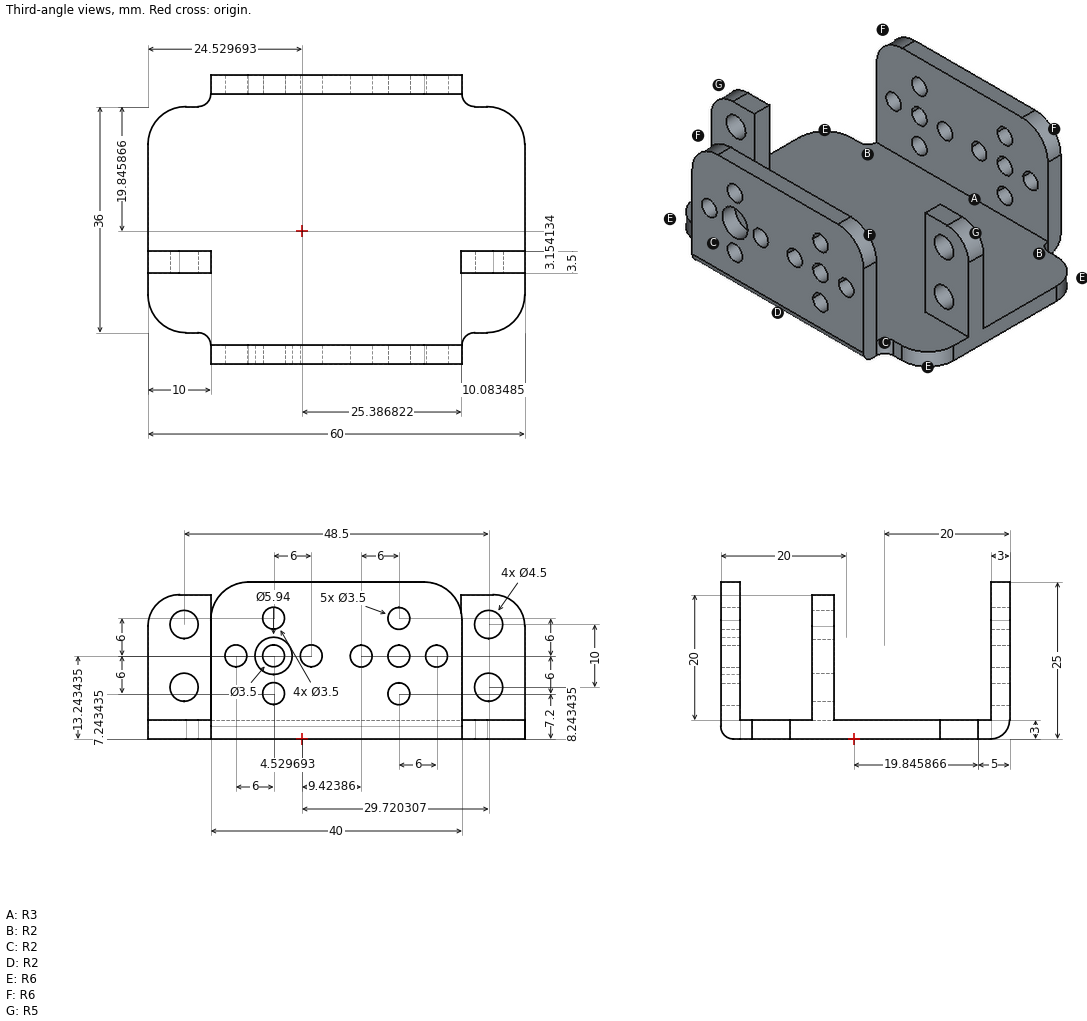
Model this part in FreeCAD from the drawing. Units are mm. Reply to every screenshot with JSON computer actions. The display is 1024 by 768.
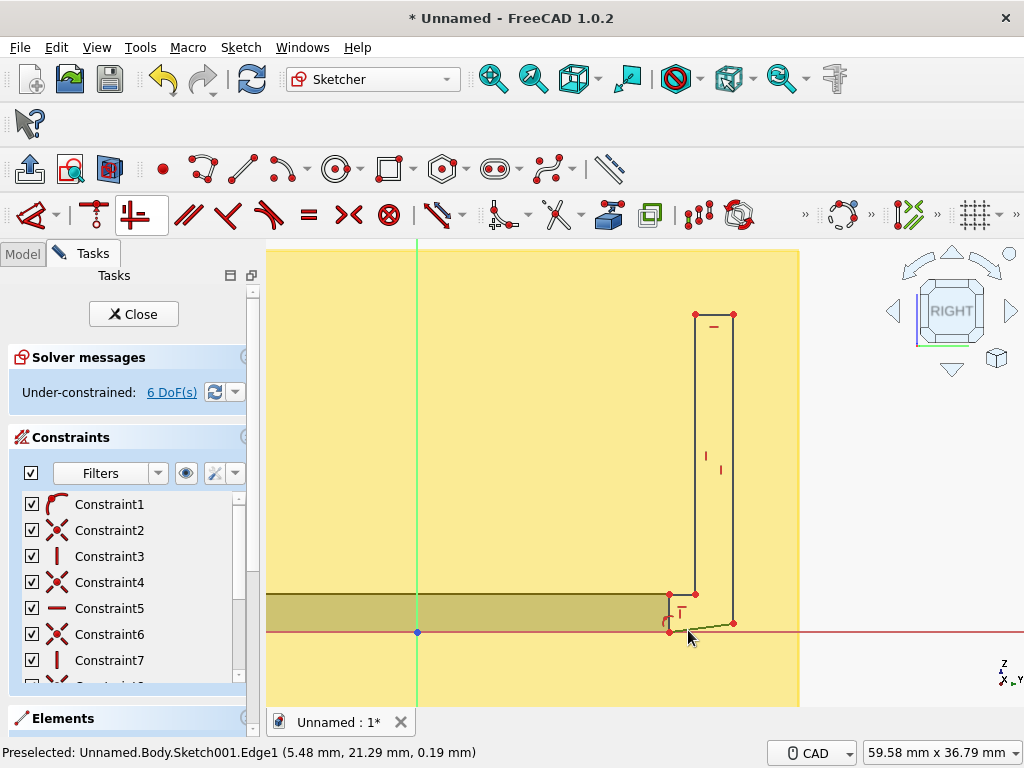
{"action": "left_click", "coordinate": [162, 216]}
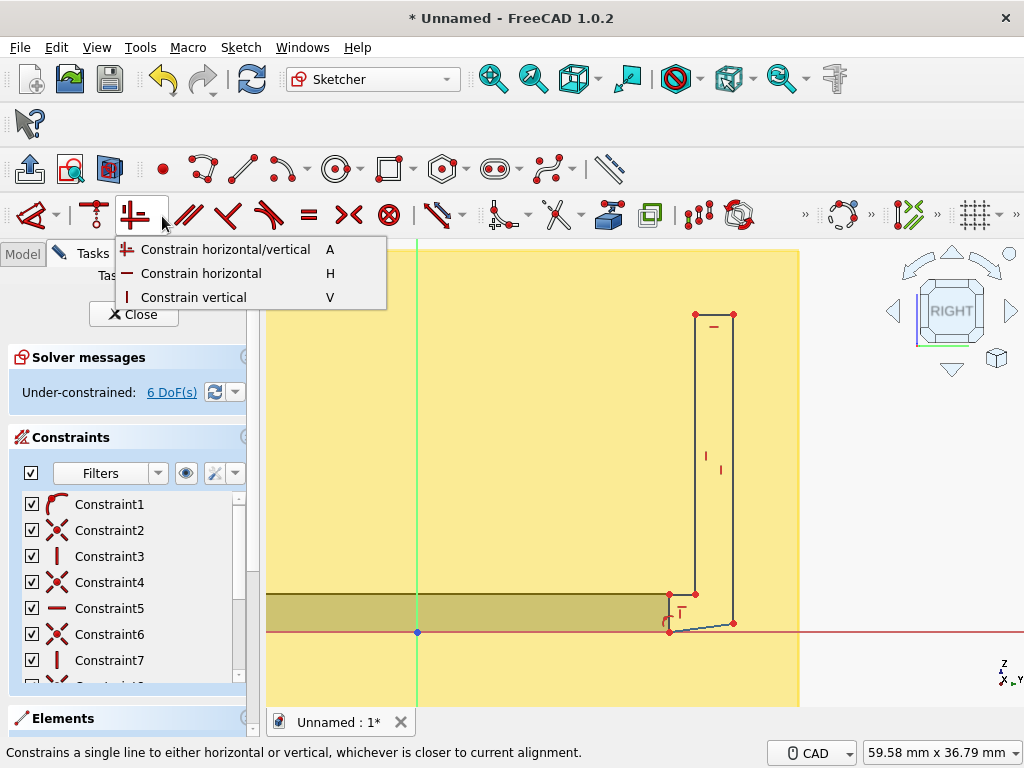
{"action": "left_click", "coordinate": [251, 273]}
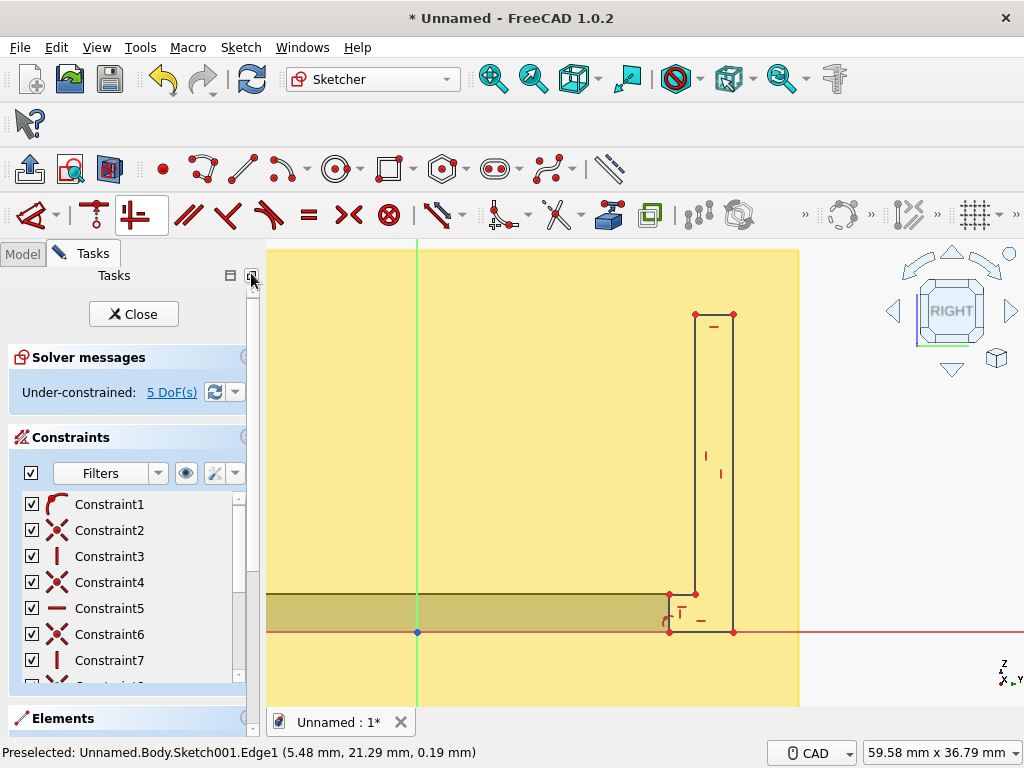
{"action": "left_click", "coordinate": [32, 216]}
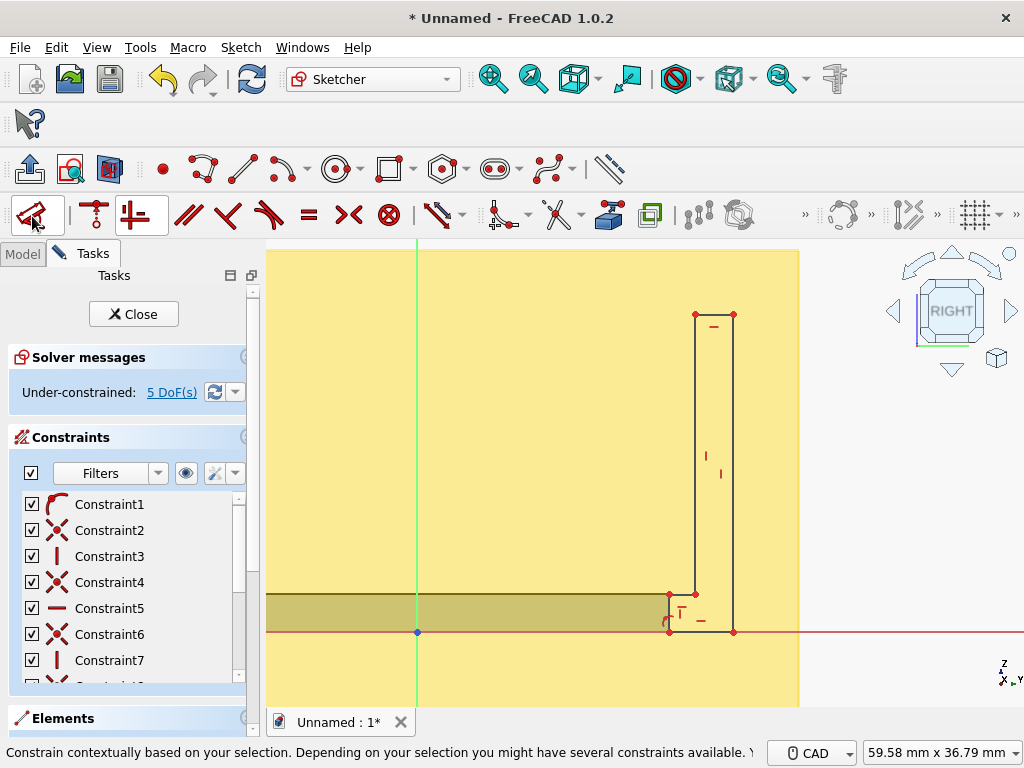
{"action": "left_click", "coordinate": [688, 632]}
{"action": "left_click", "coordinate": [701, 666]}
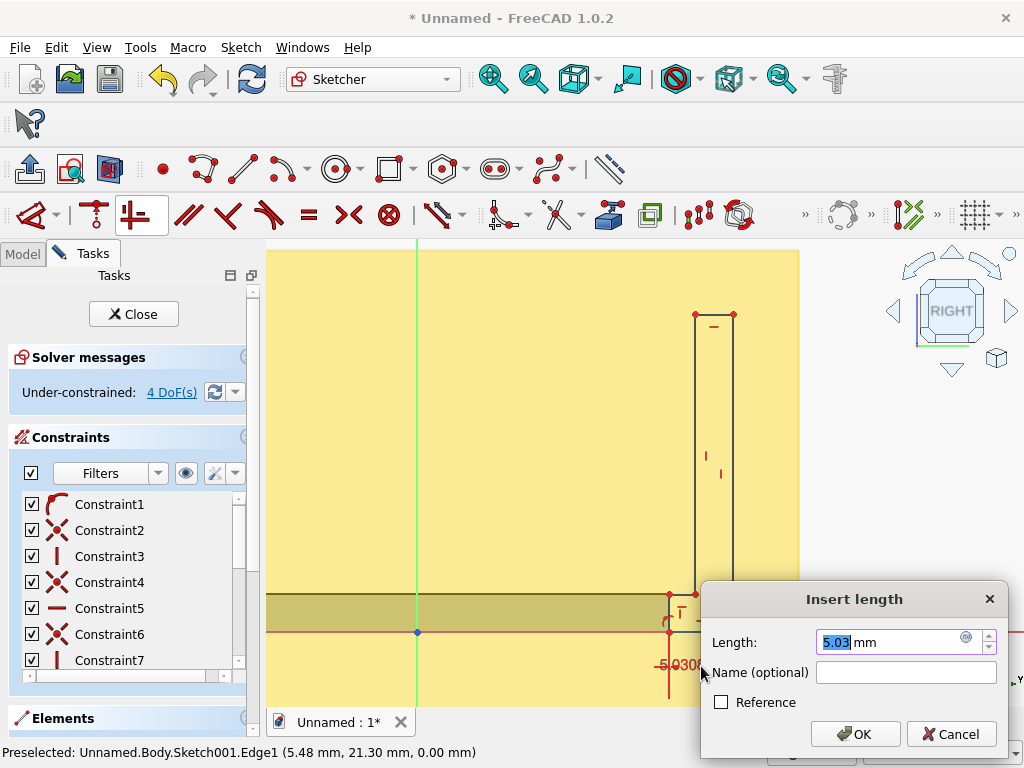
{"action": "type", "text": "5"}
{"action": "key", "text": "Return"}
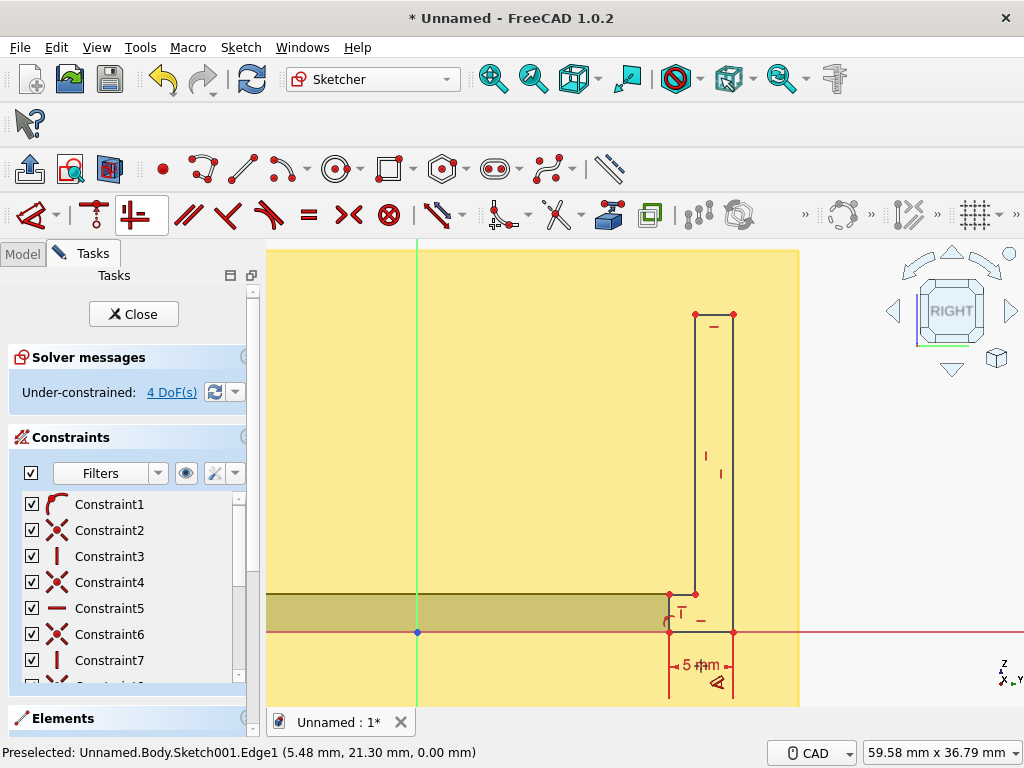
{"action": "left_click", "coordinate": [722, 315]}
{"action": "left_click", "coordinate": [714, 281]}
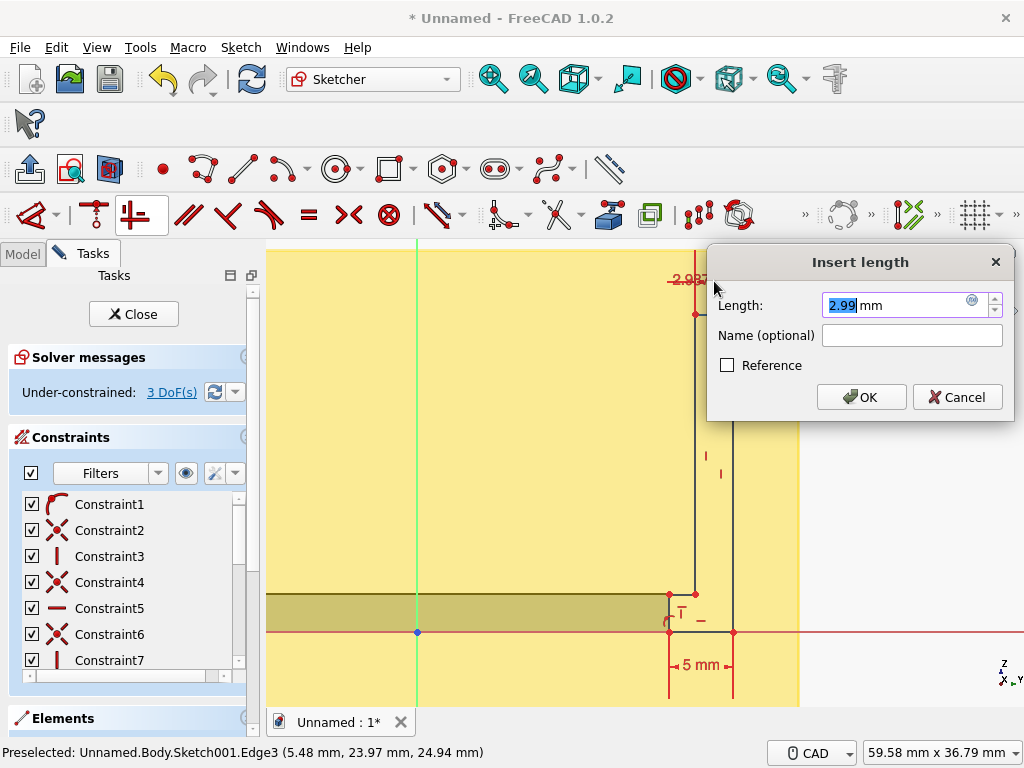
{"action": "type", "text": "3"}
{"action": "key", "text": "Return"}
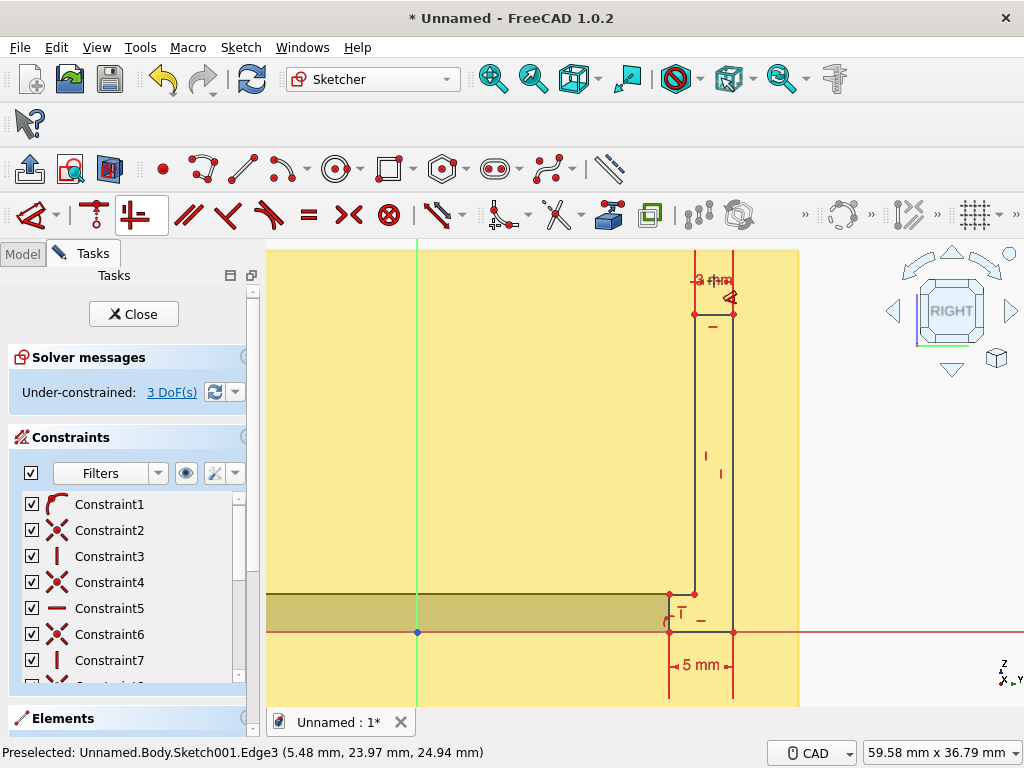
{"action": "scroll", "coordinate": [669, 606], "scroll_direction": "up", "scroll_amount": 2}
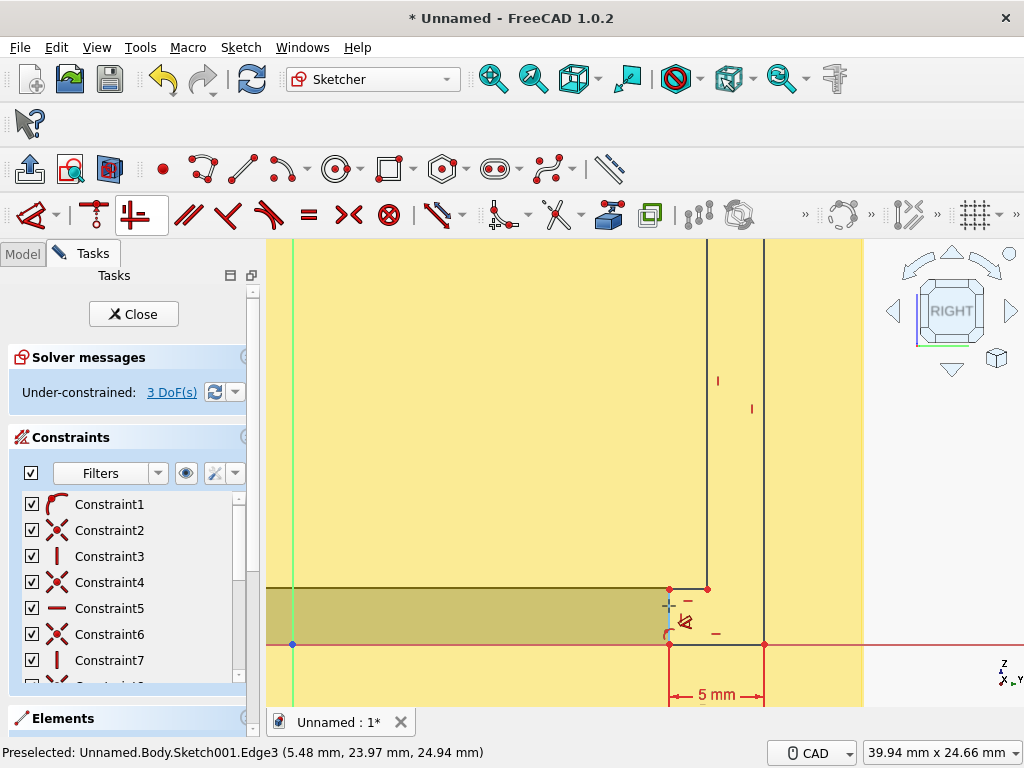
{"action": "left_click", "coordinate": [669, 606]}
{"action": "left_click", "coordinate": [703, 617]}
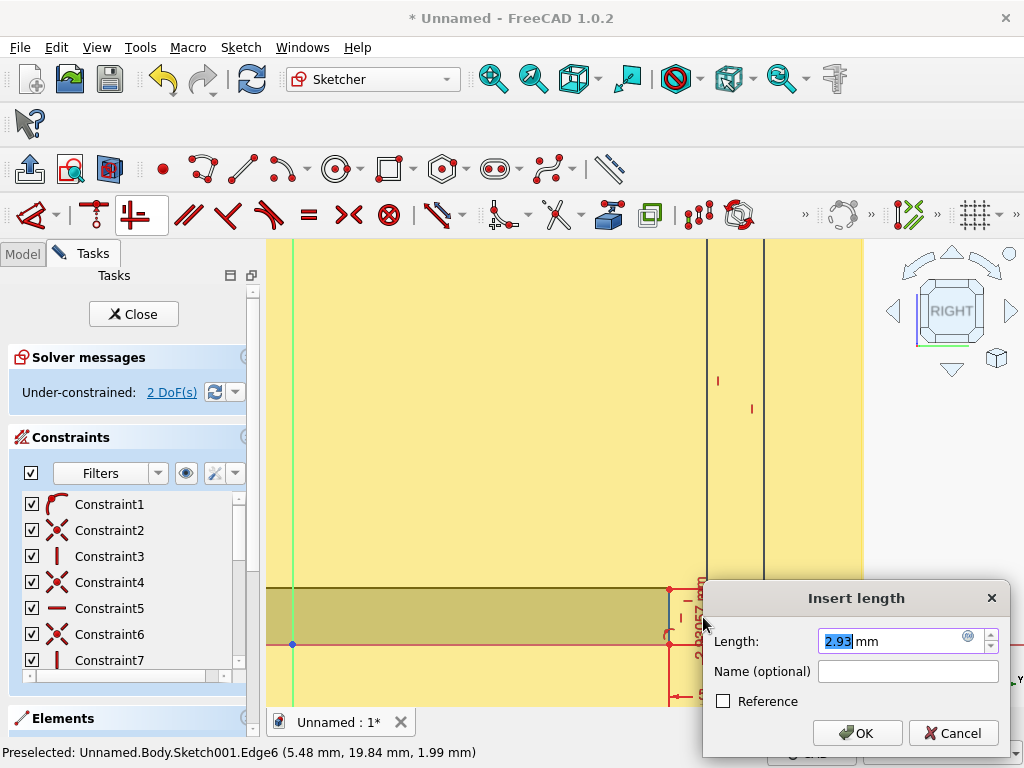
{"action": "type", "text": "3"}
{"action": "key", "text": "Return"}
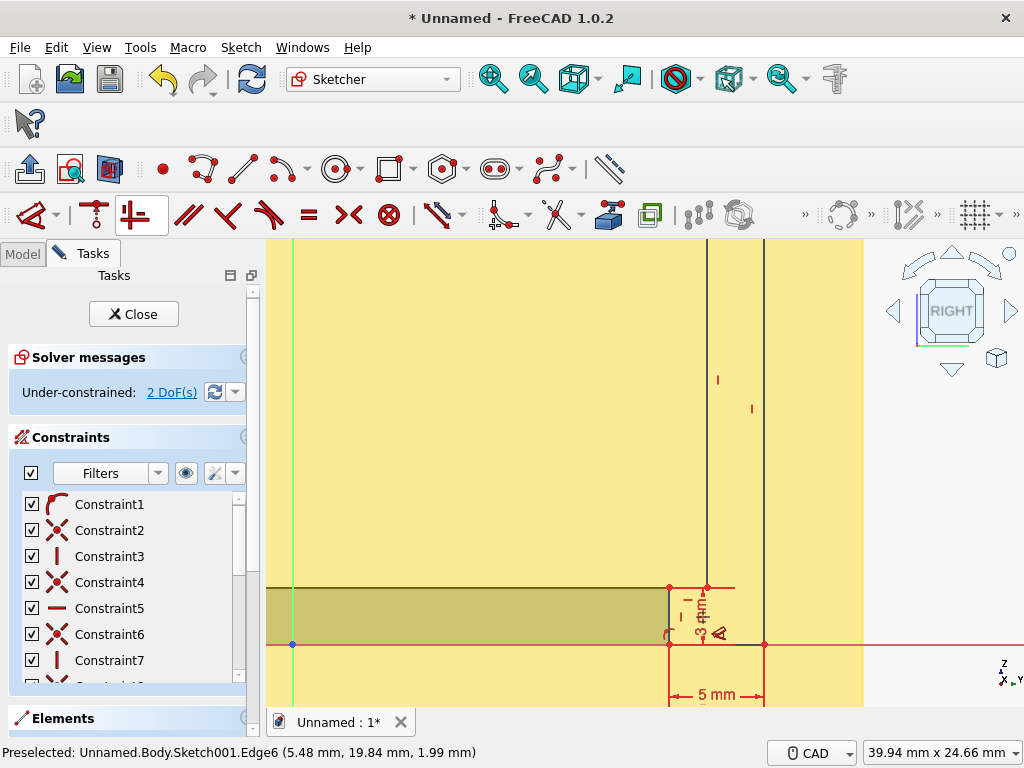
{"action": "left_click", "coordinate": [764, 503]}
{"action": "left_click", "coordinate": [798, 456]}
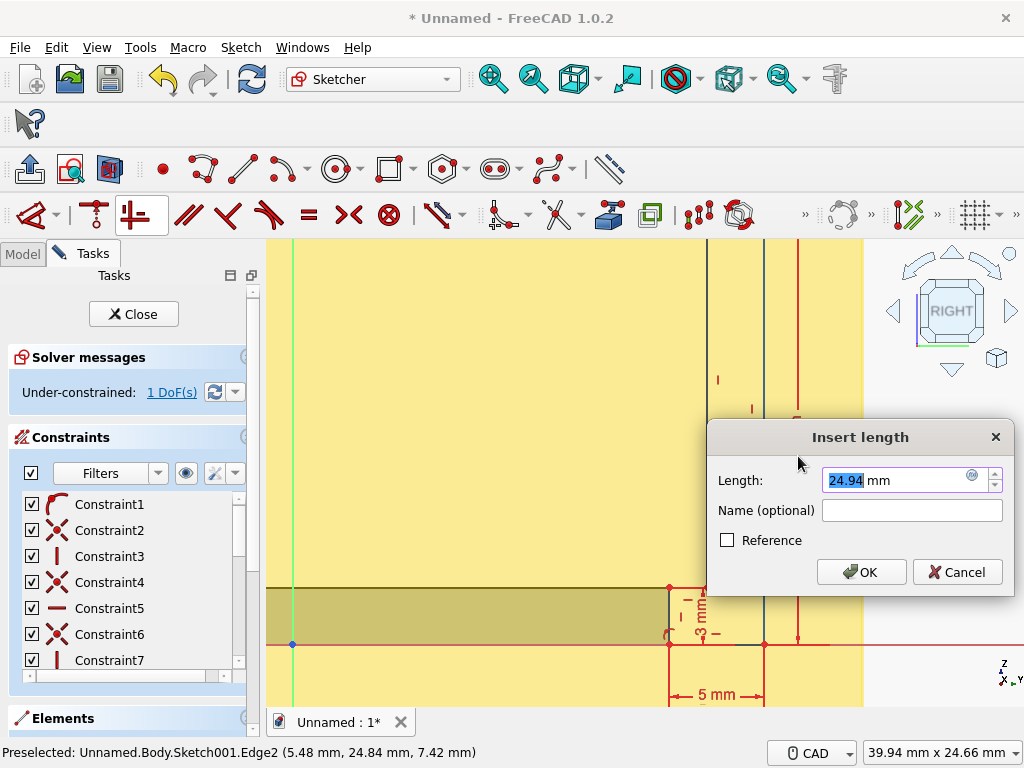
{"action": "type", "text": "25"}
{"action": "key", "text": "Return"}